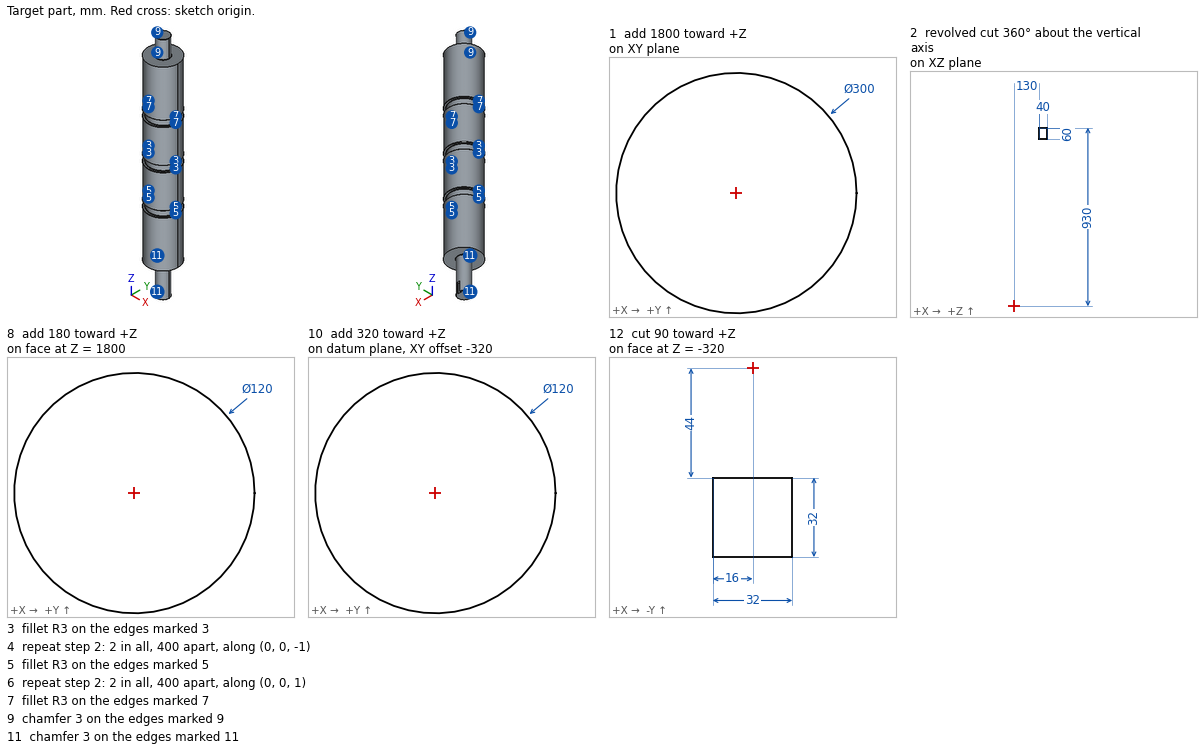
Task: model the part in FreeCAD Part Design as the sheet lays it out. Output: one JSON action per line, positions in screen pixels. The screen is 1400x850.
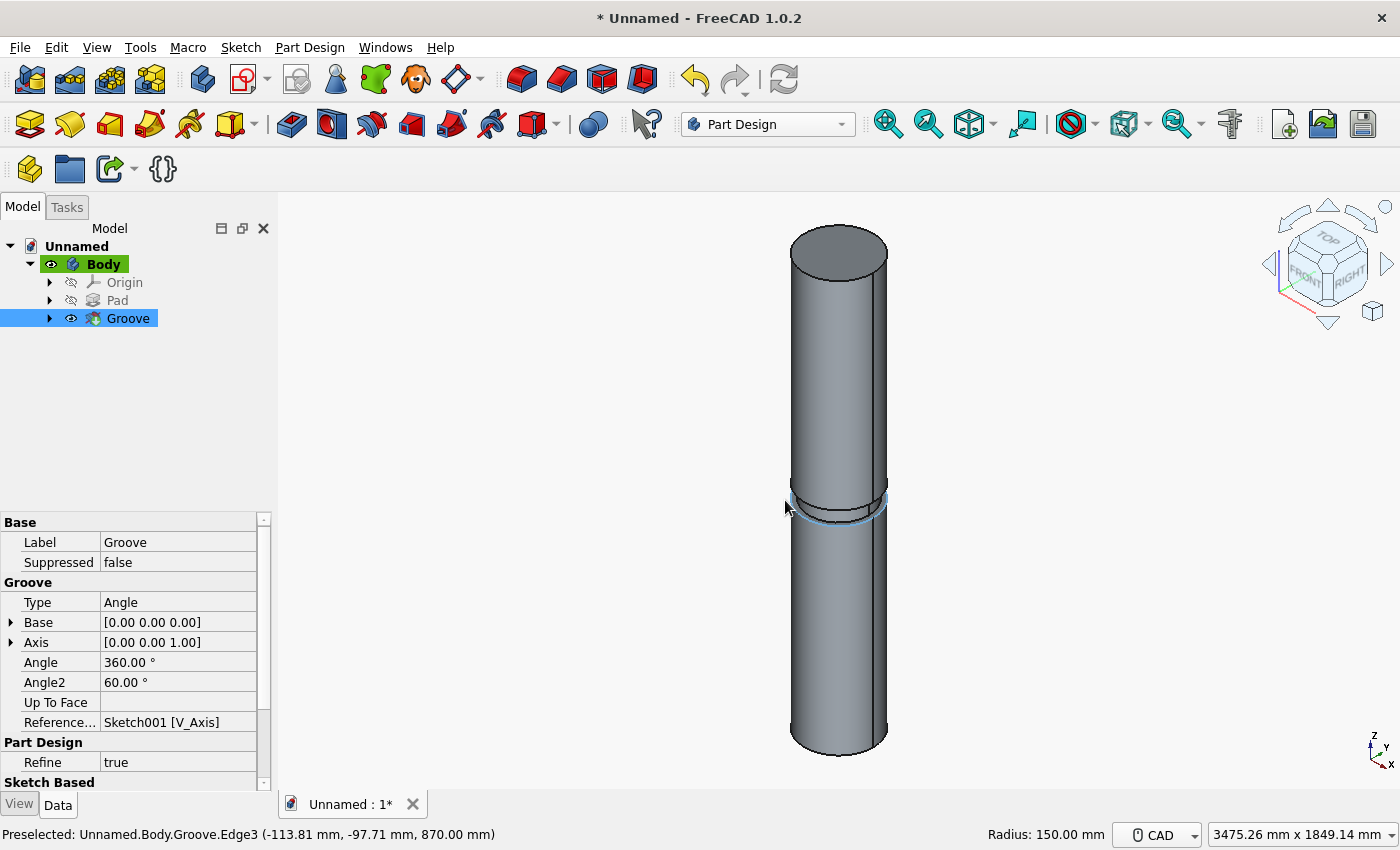
{"action": "key", "text": "2"}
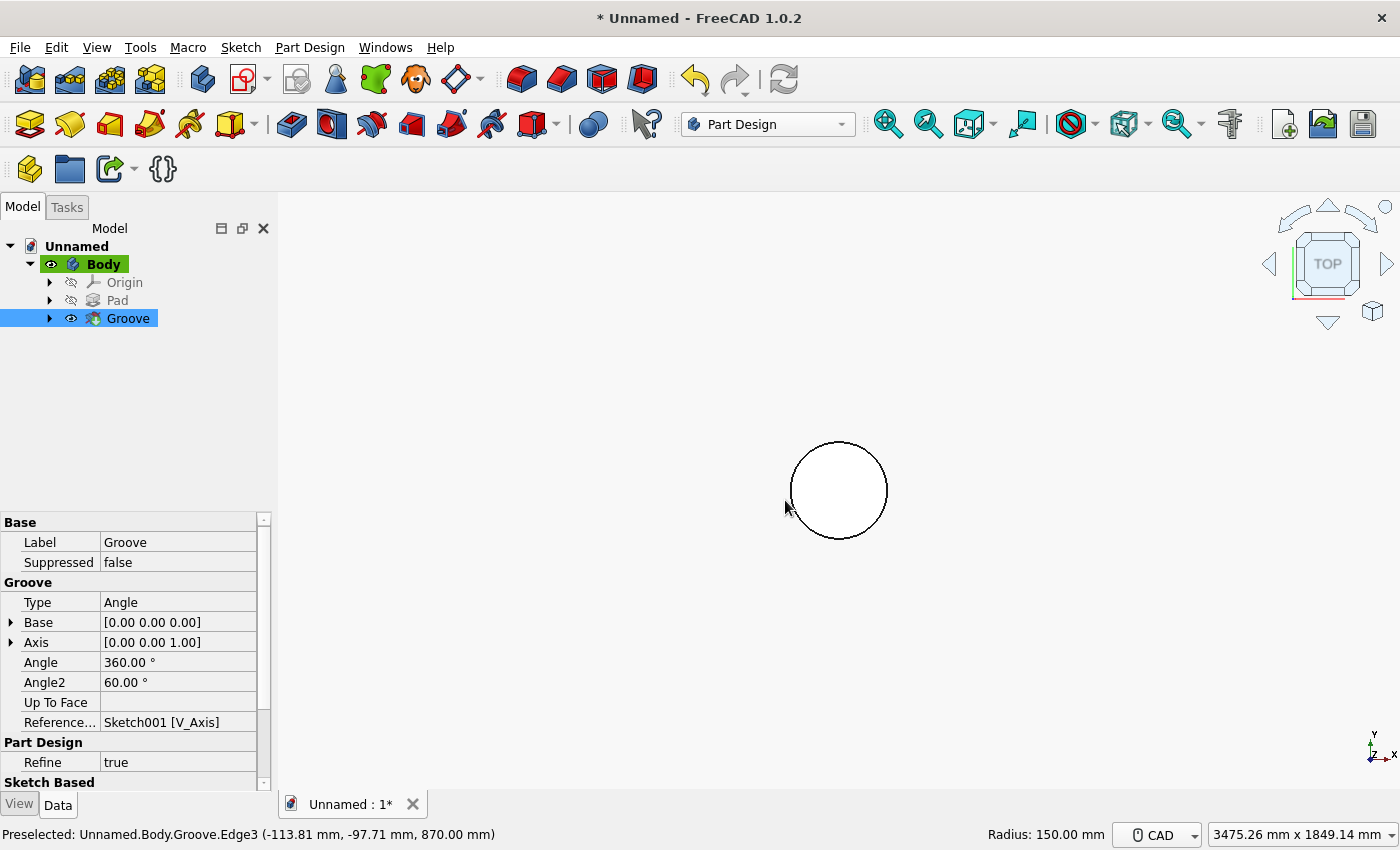
{"action": "left_click", "coordinate": [890, 124]}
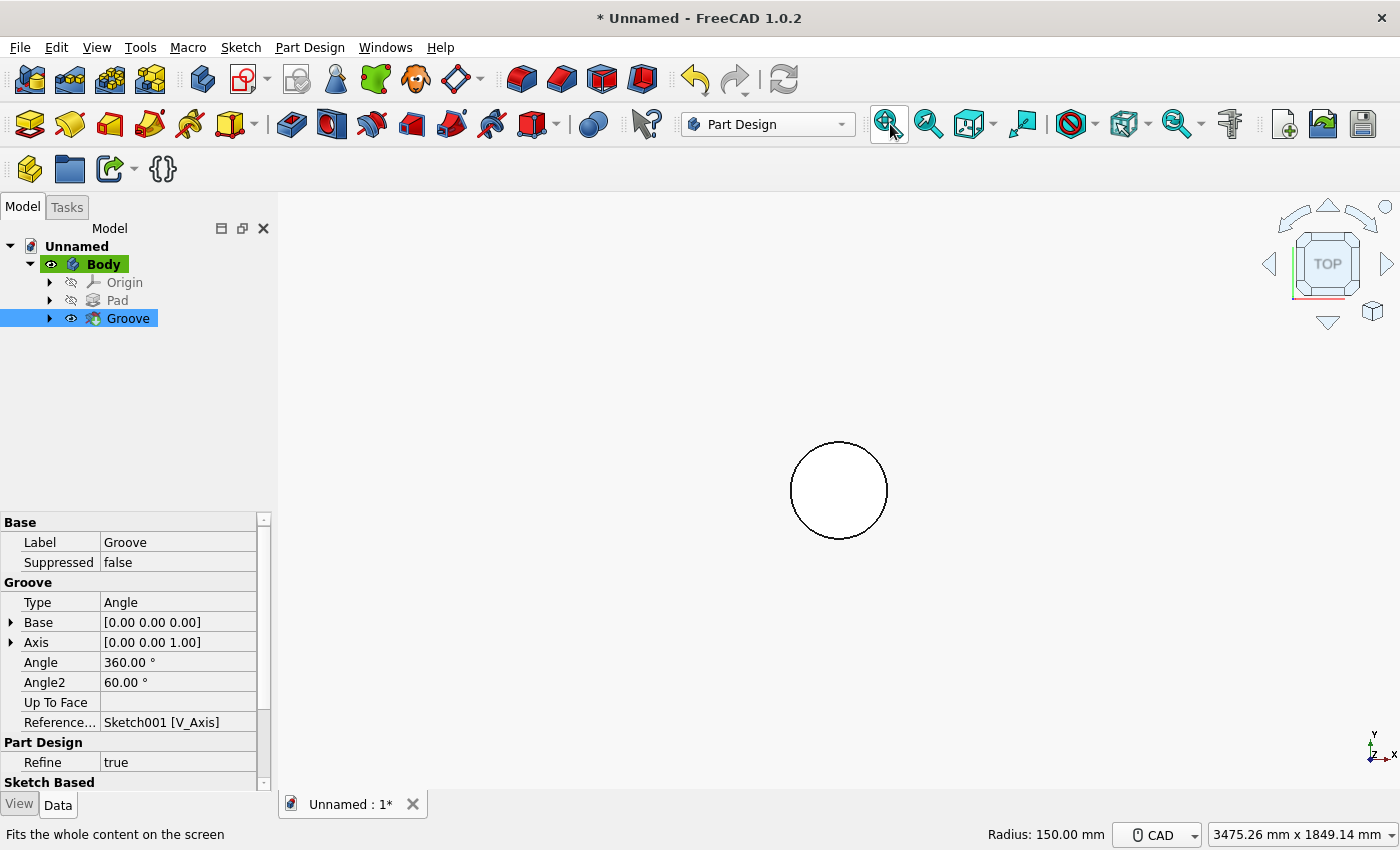
{"action": "key", "text": "1"}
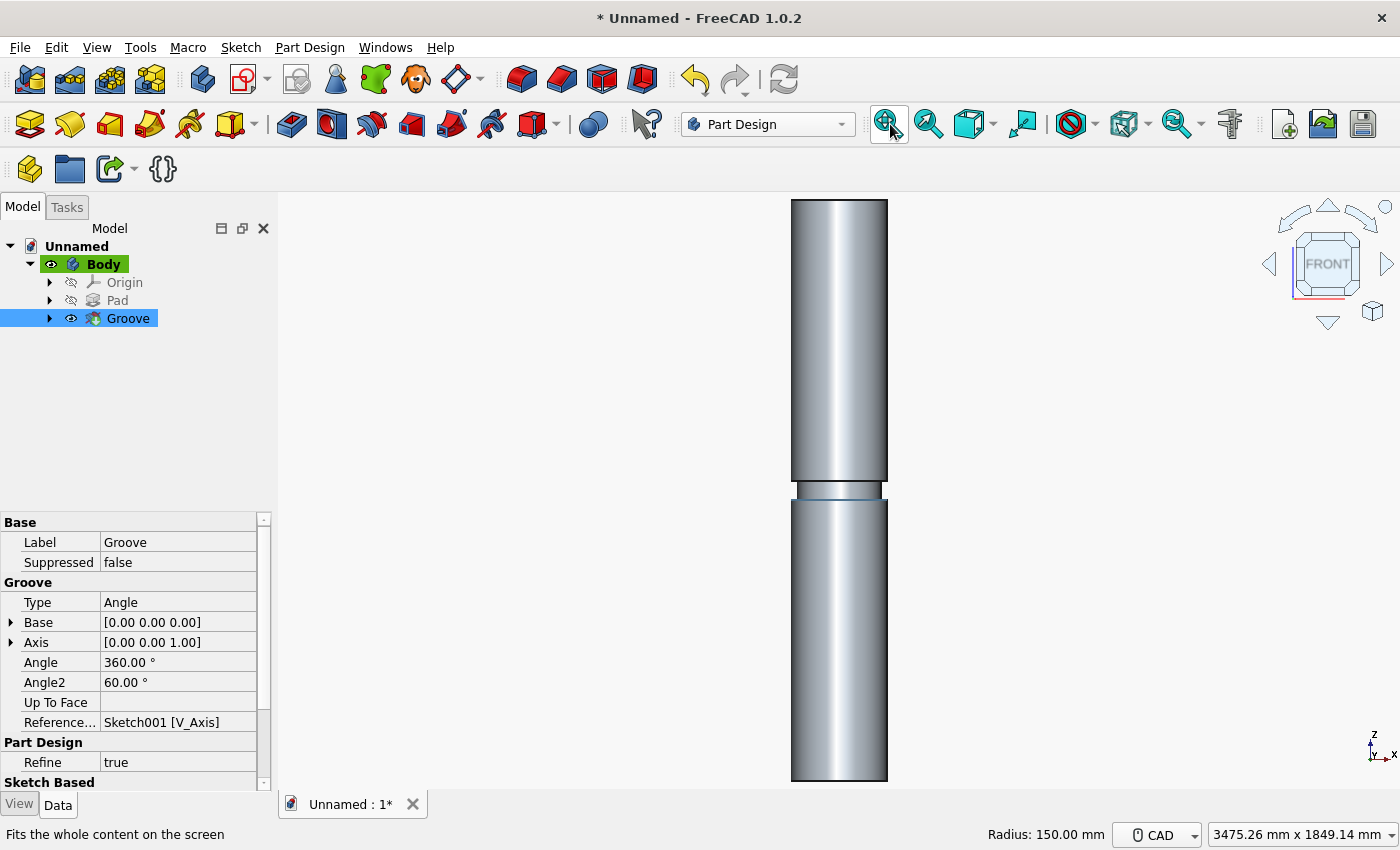
{"action": "left_click", "coordinate": [800, 480], "text": "ctrl"}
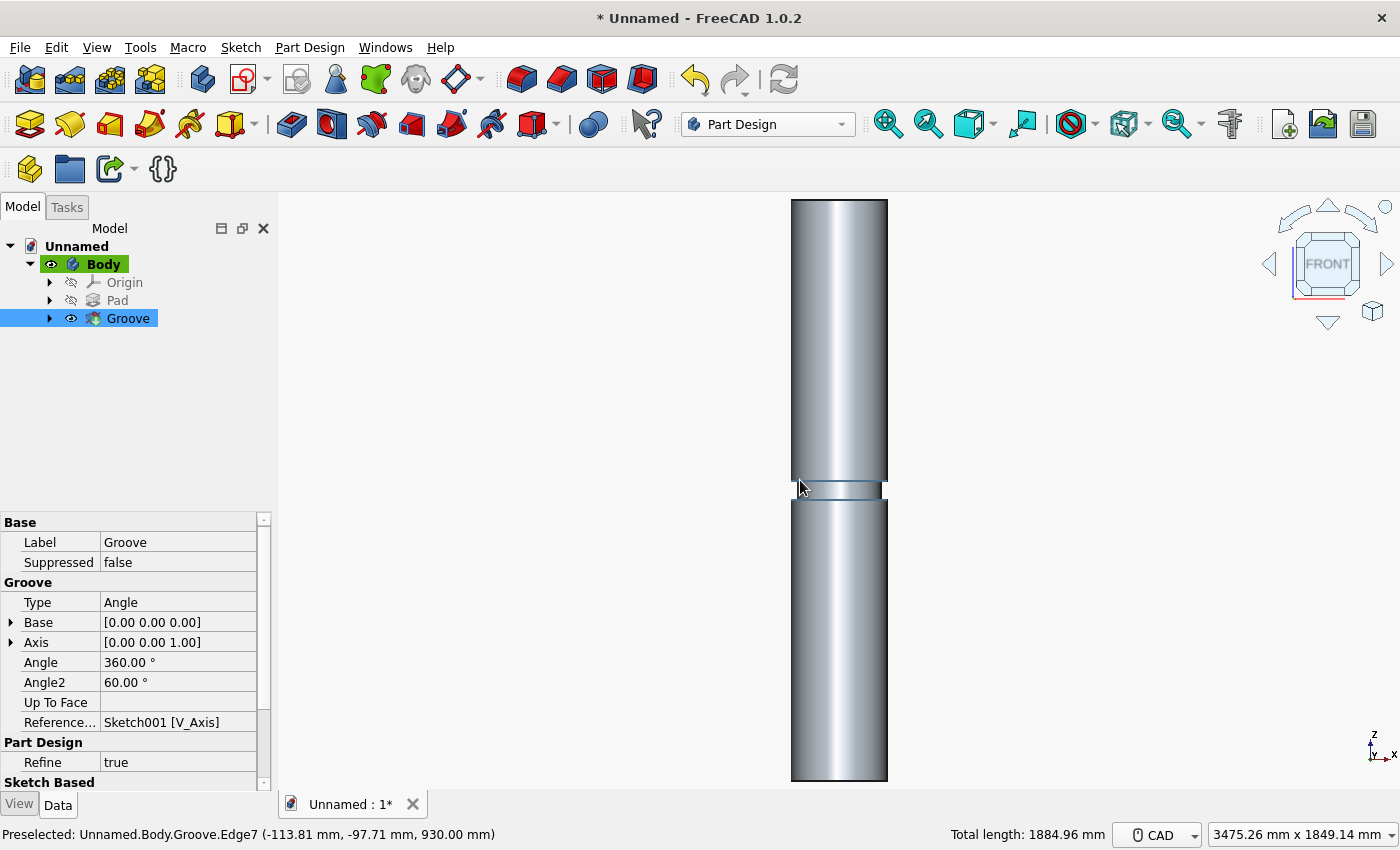
{"action": "key", "text": "3"}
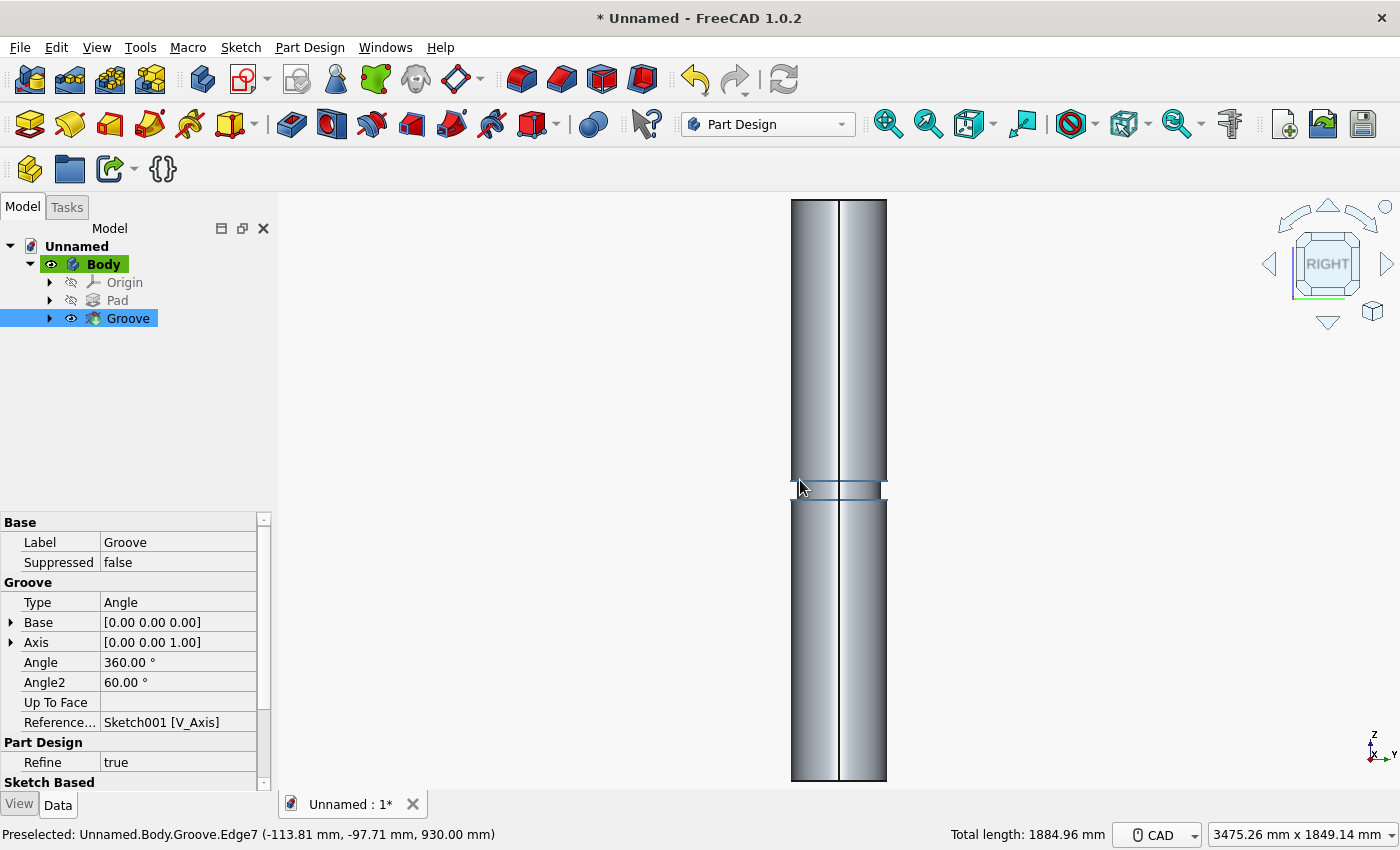
{"action": "key", "text": "5"}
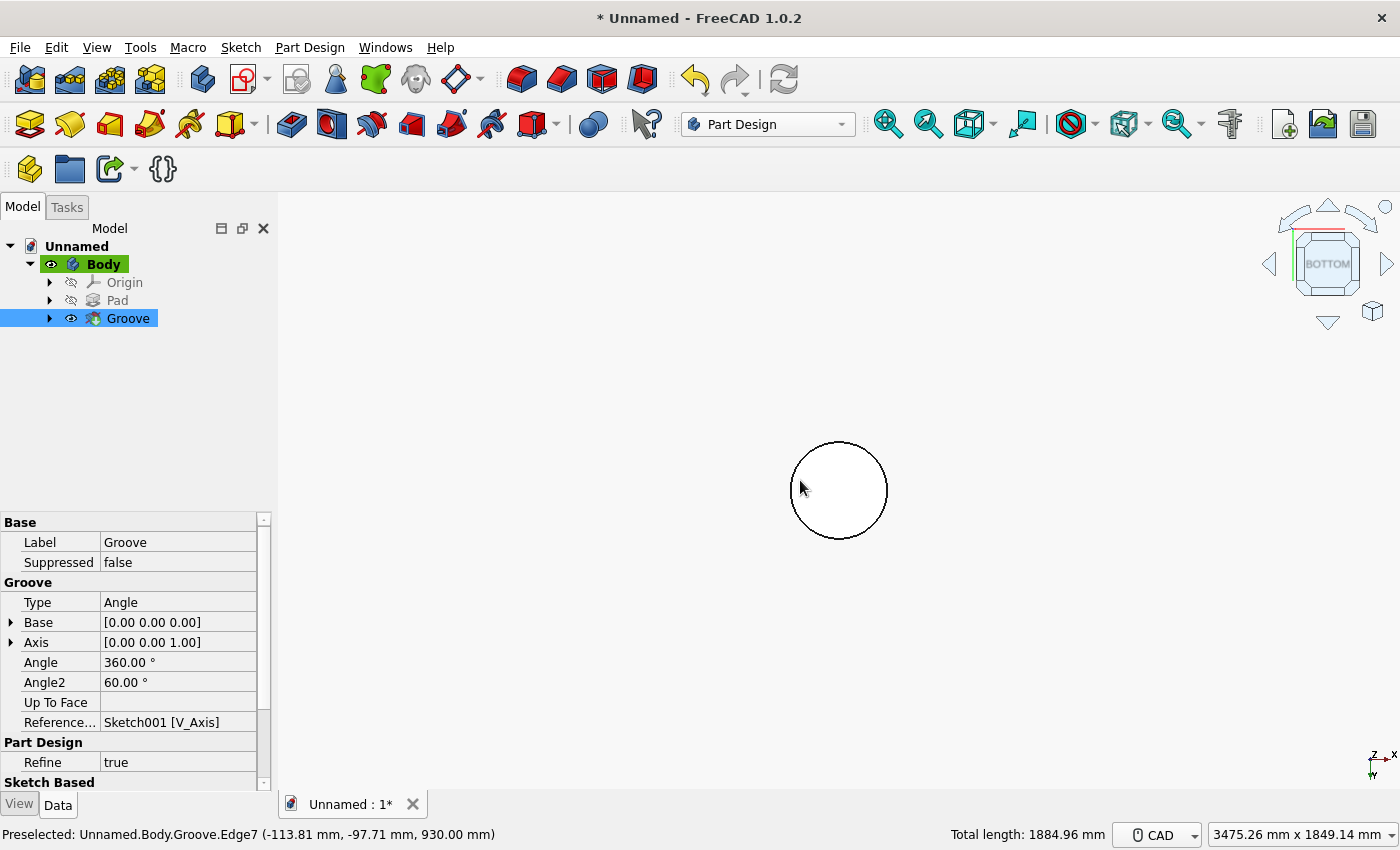
{"action": "left_click", "coordinate": [890, 124]}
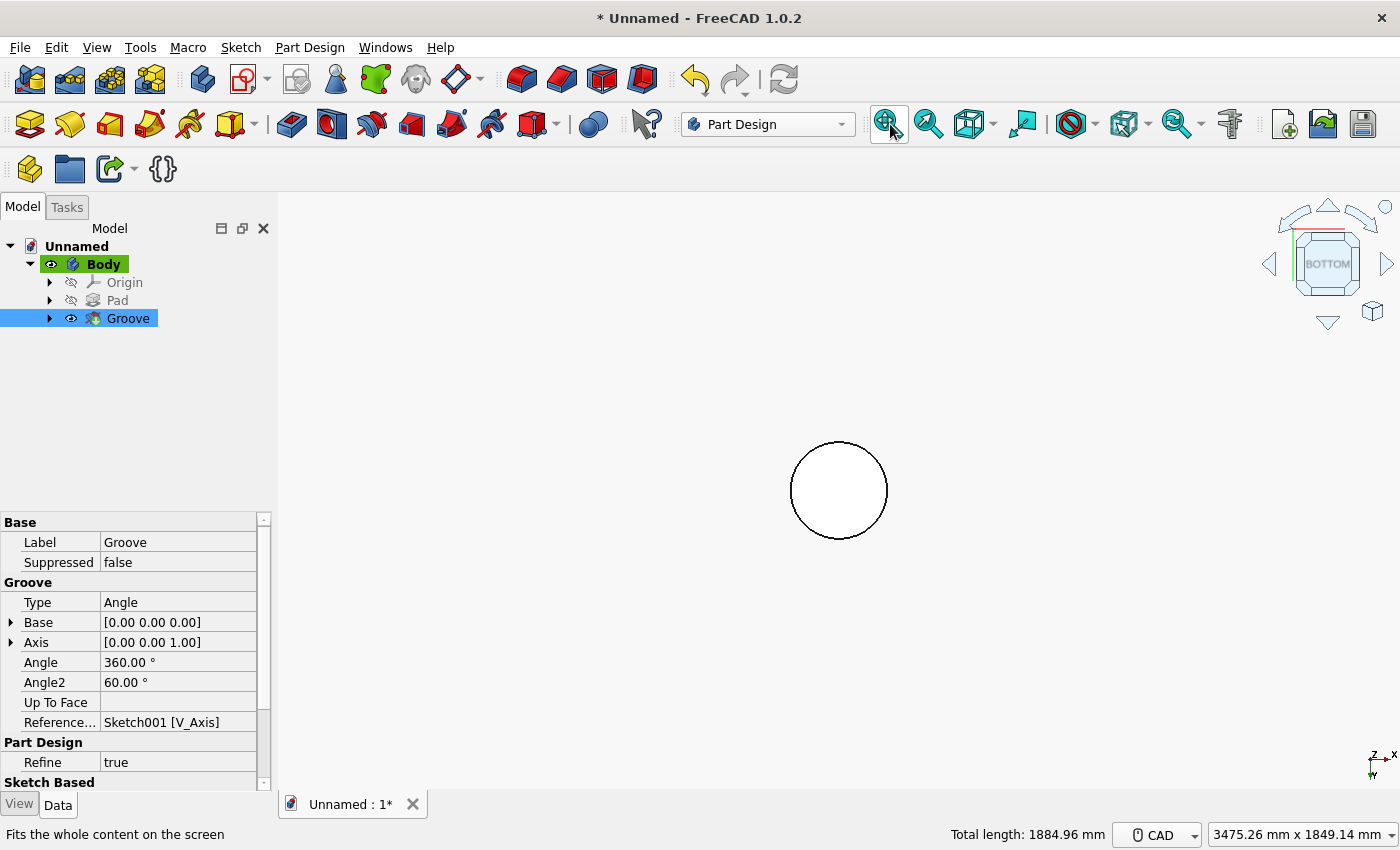
{"action": "key", "text": "4"}